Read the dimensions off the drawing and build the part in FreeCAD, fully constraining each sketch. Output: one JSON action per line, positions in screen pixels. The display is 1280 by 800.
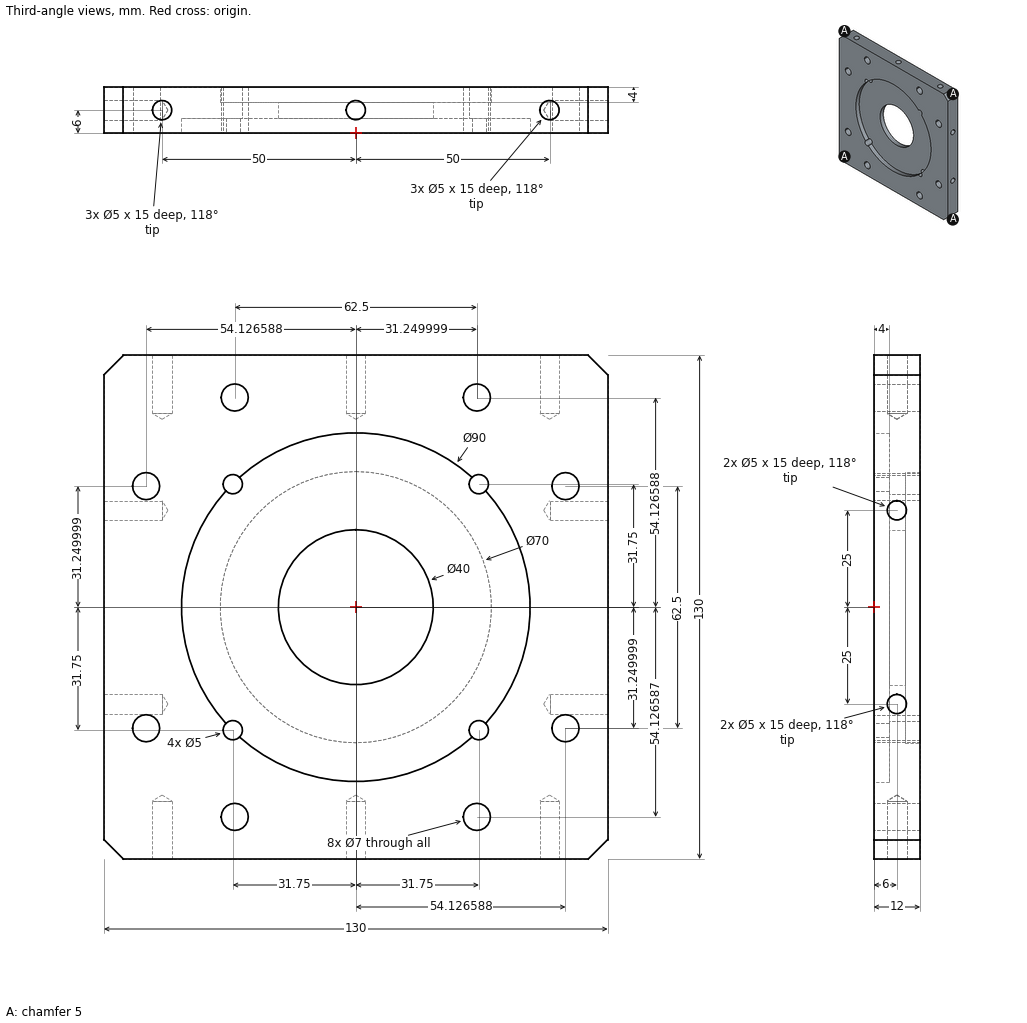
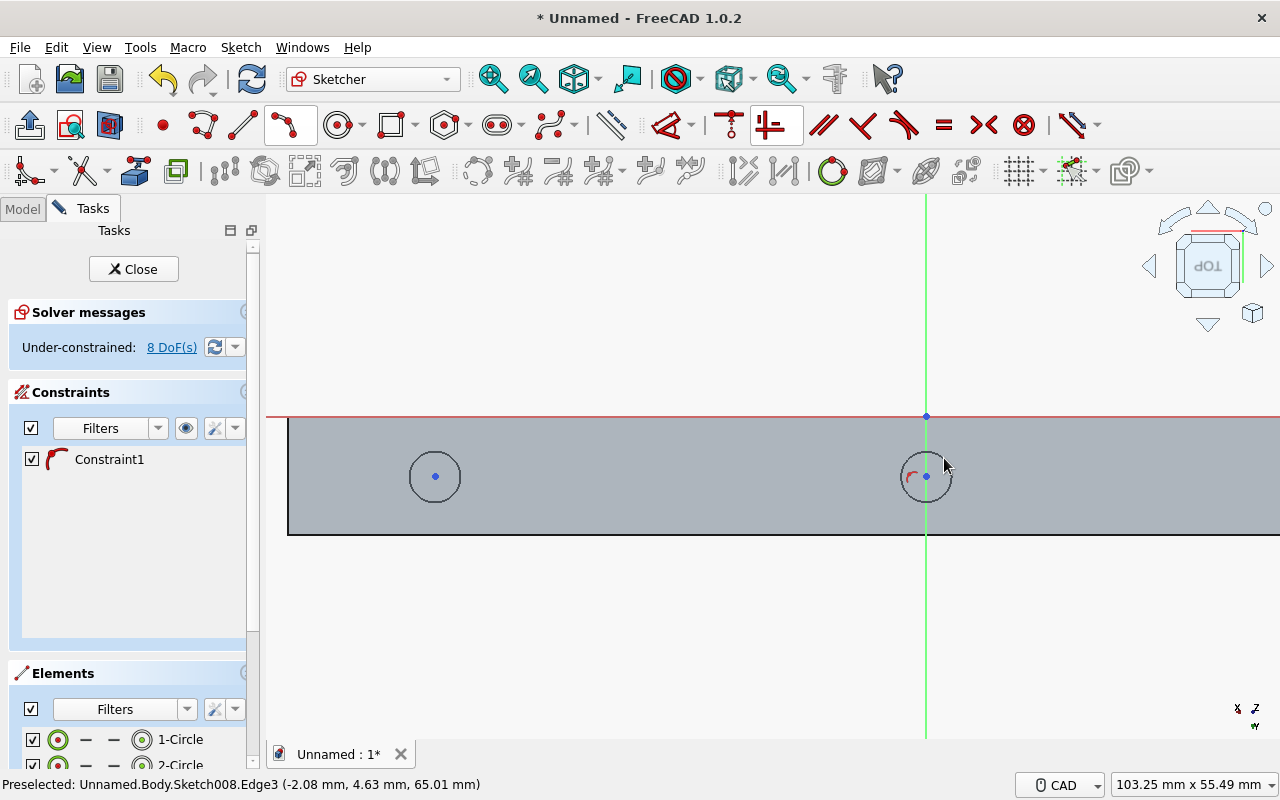
{"action": "scroll", "coordinate": [435, 476], "scroll_direction": "down", "scroll_amount": 3}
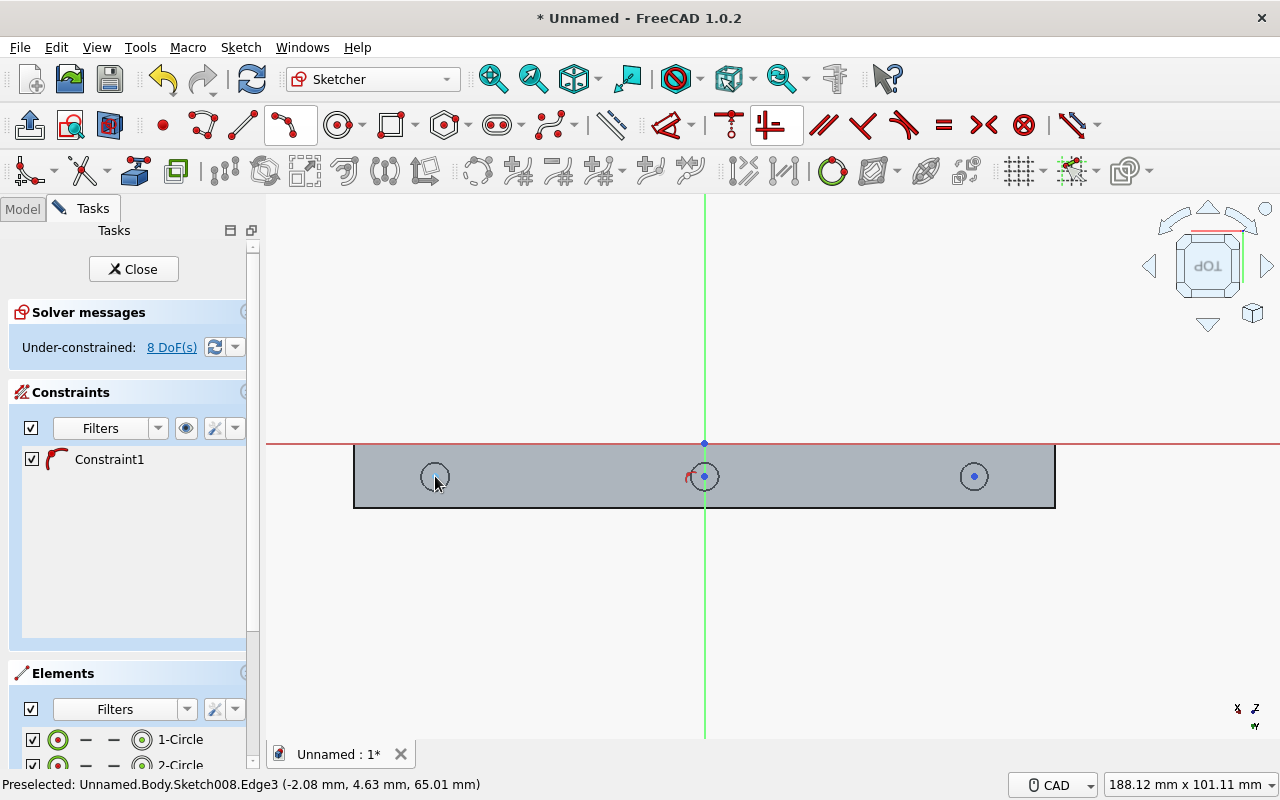
{"action": "left_click", "coordinate": [984, 467]}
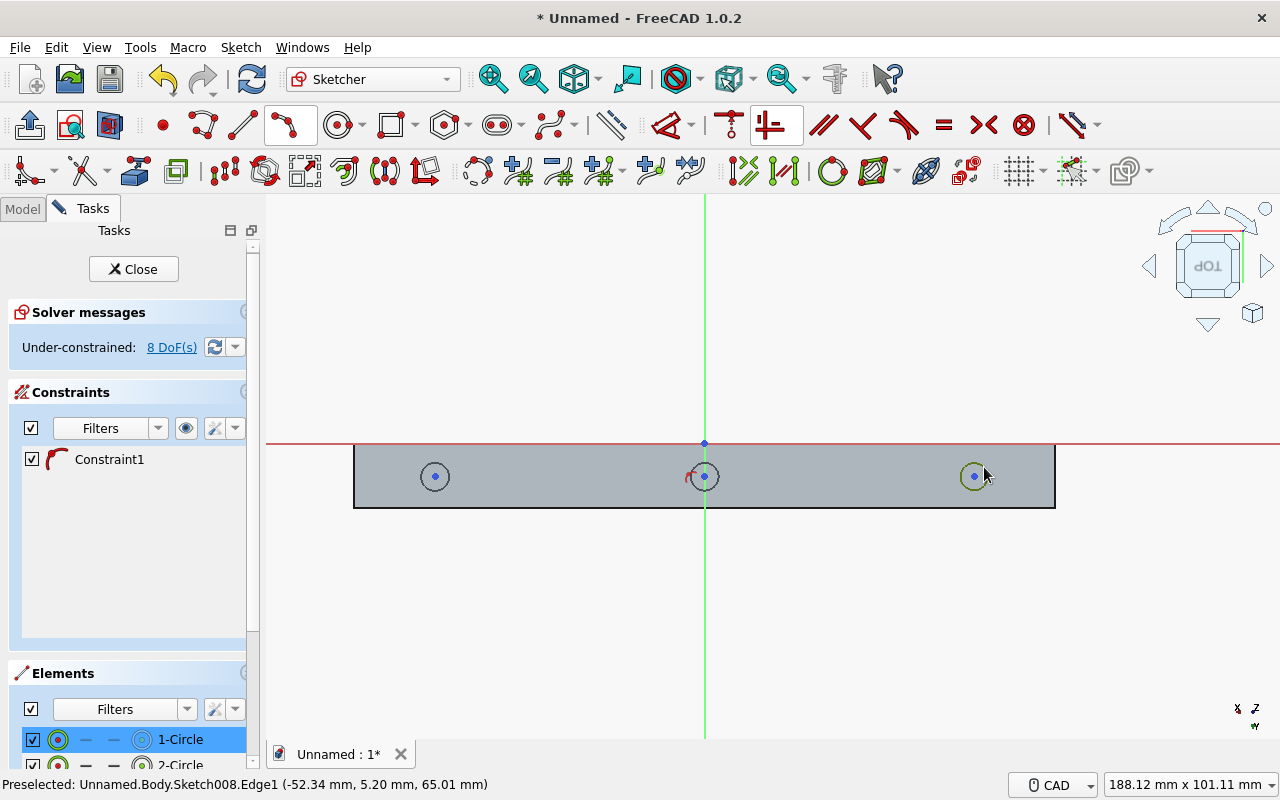
{"action": "left_click", "coordinate": [445, 467]}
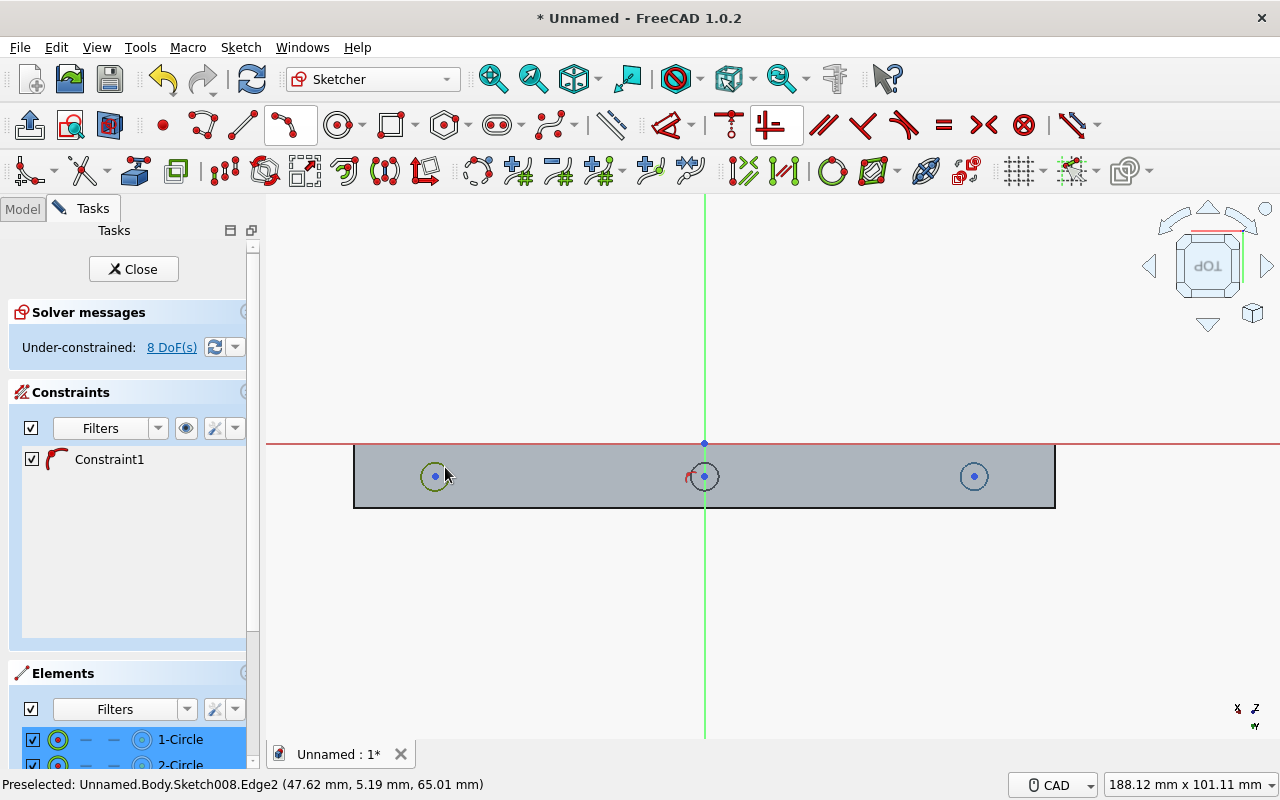
{"action": "scroll", "coordinate": [714, 467], "scroll_direction": "up", "scroll_amount": 2}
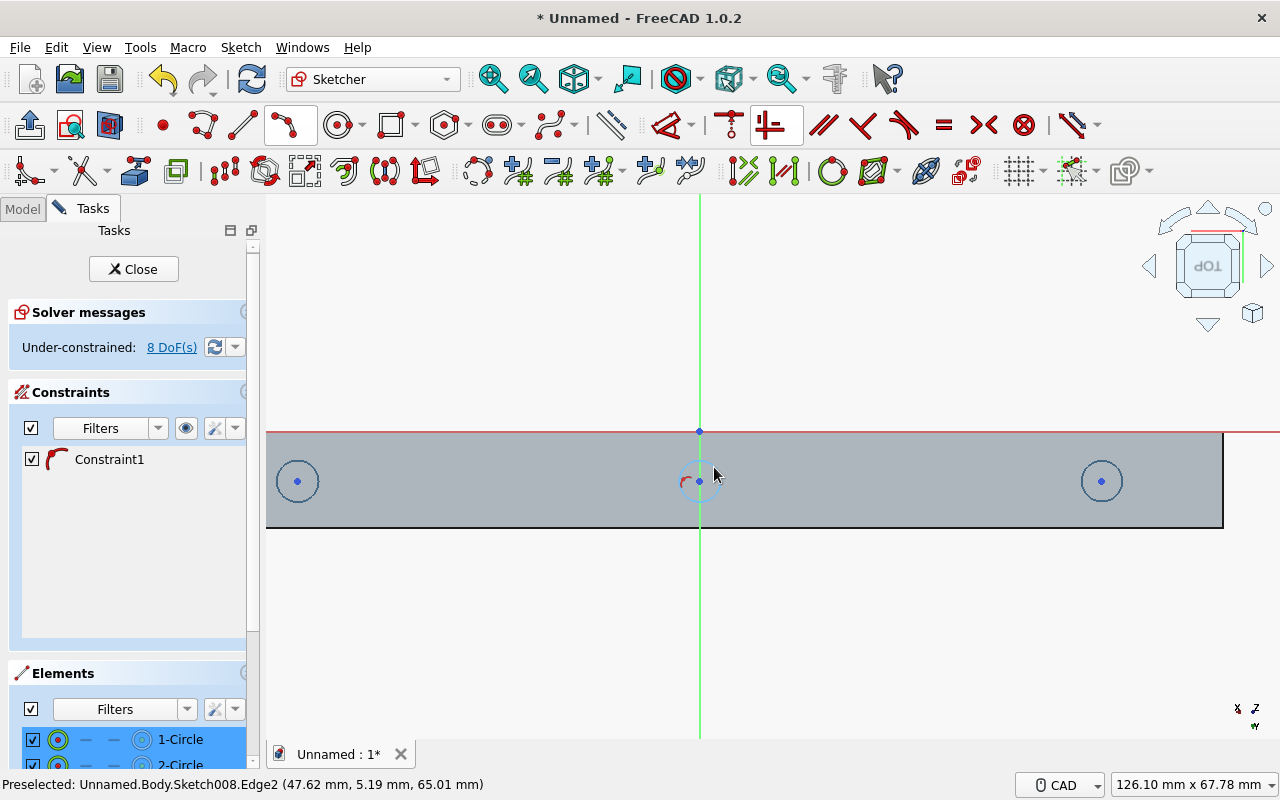
{"action": "left_click", "coordinate": [715, 467]}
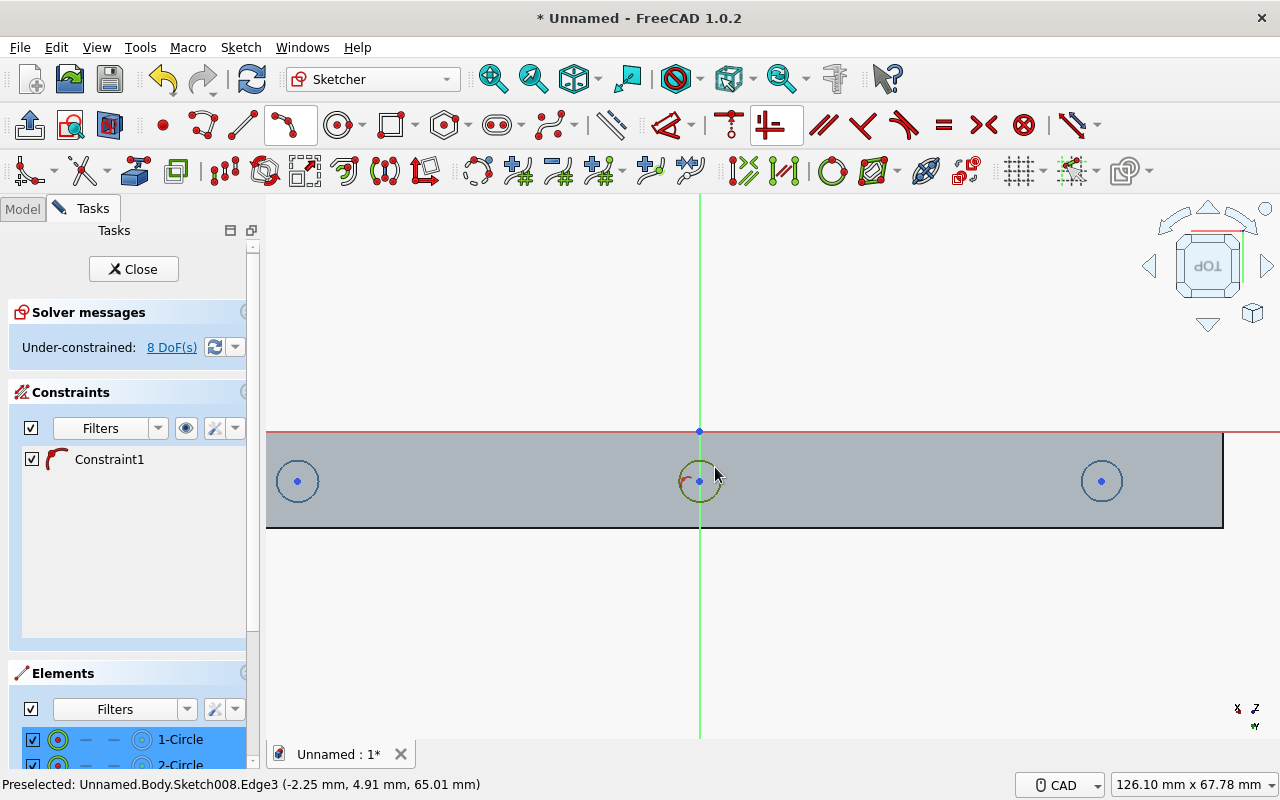
{"action": "key", "text": "e"}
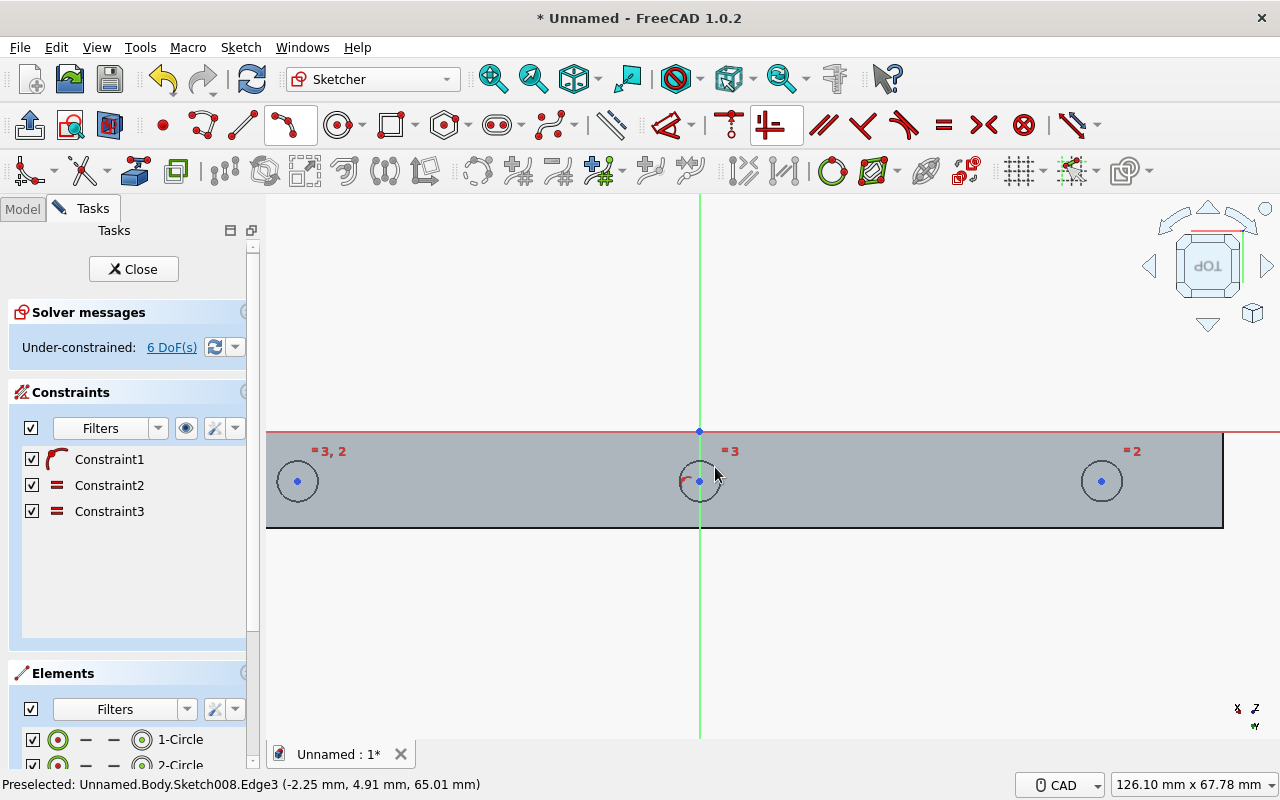
{"action": "left_click", "coordinate": [1102, 481]}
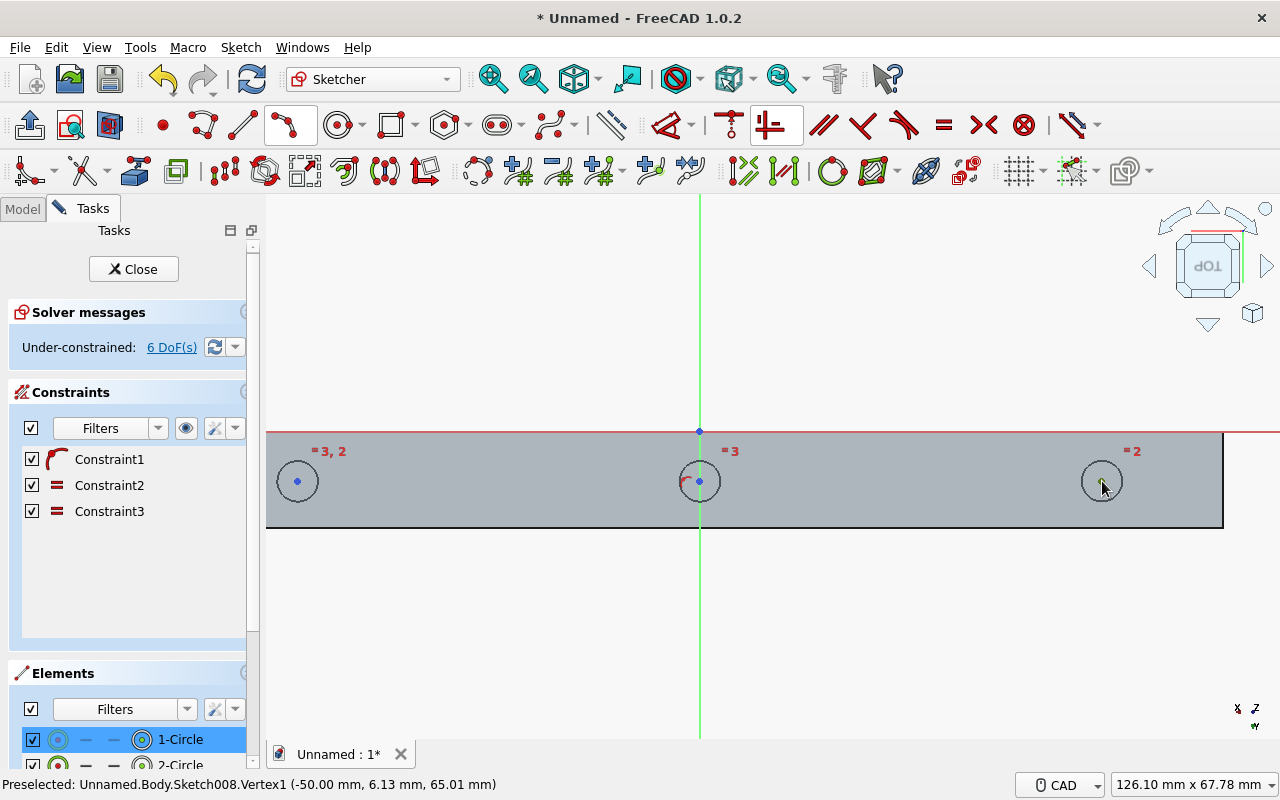
{"action": "left_click", "coordinate": [298, 481]}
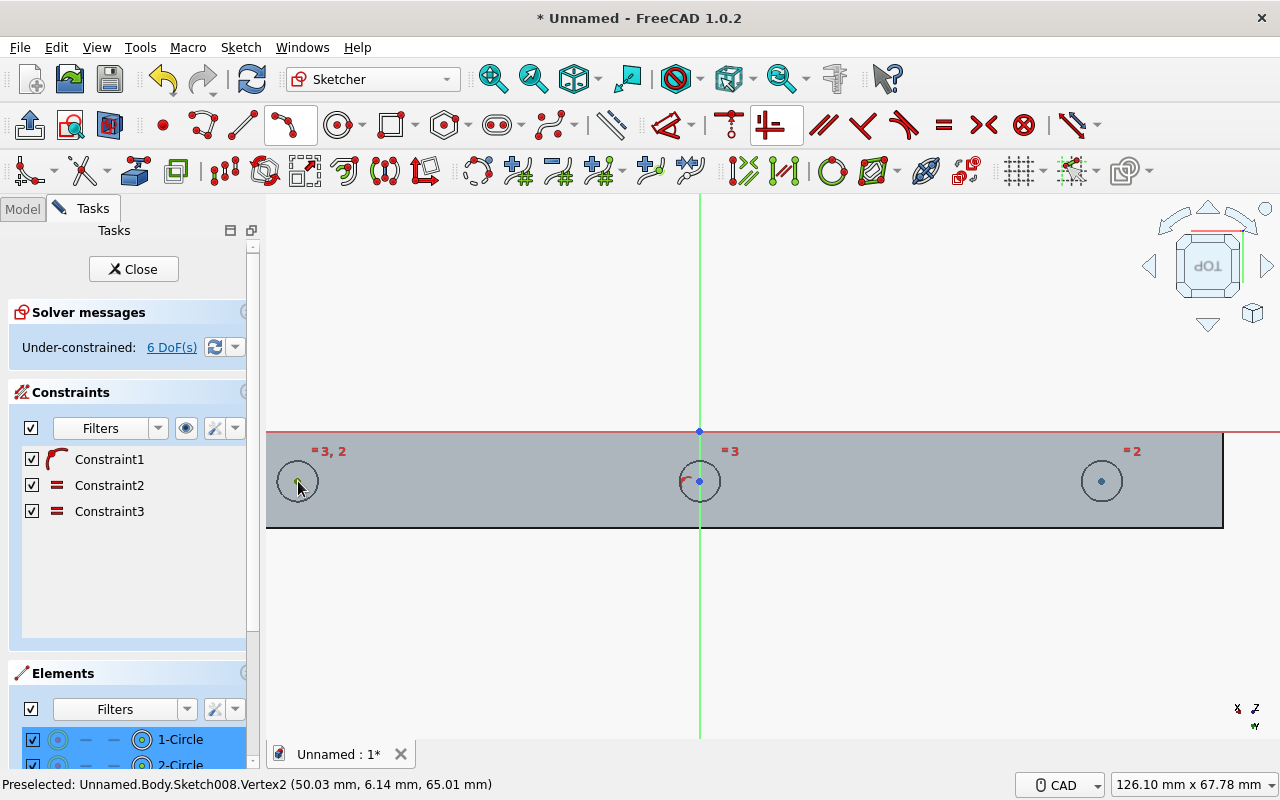
{"action": "left_click", "coordinate": [798, 126]}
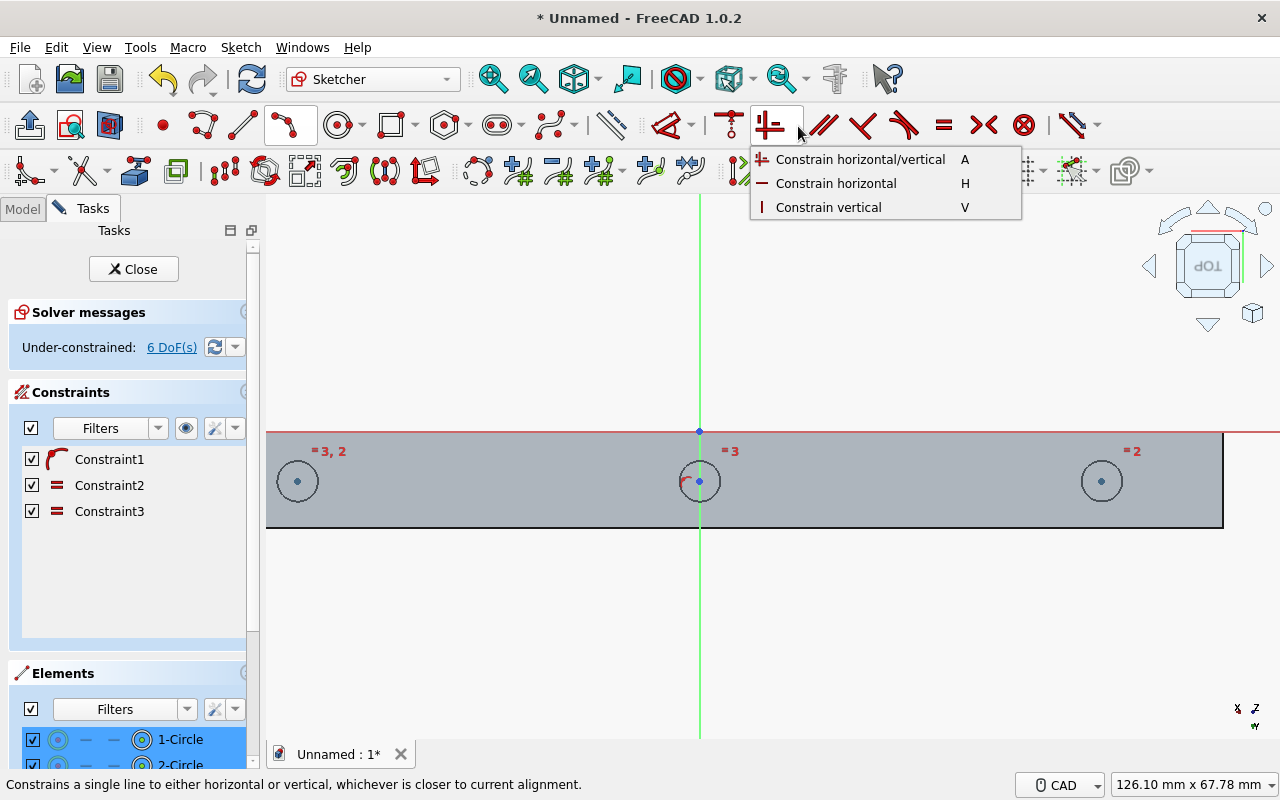
{"action": "left_click", "coordinate": [886, 183]}